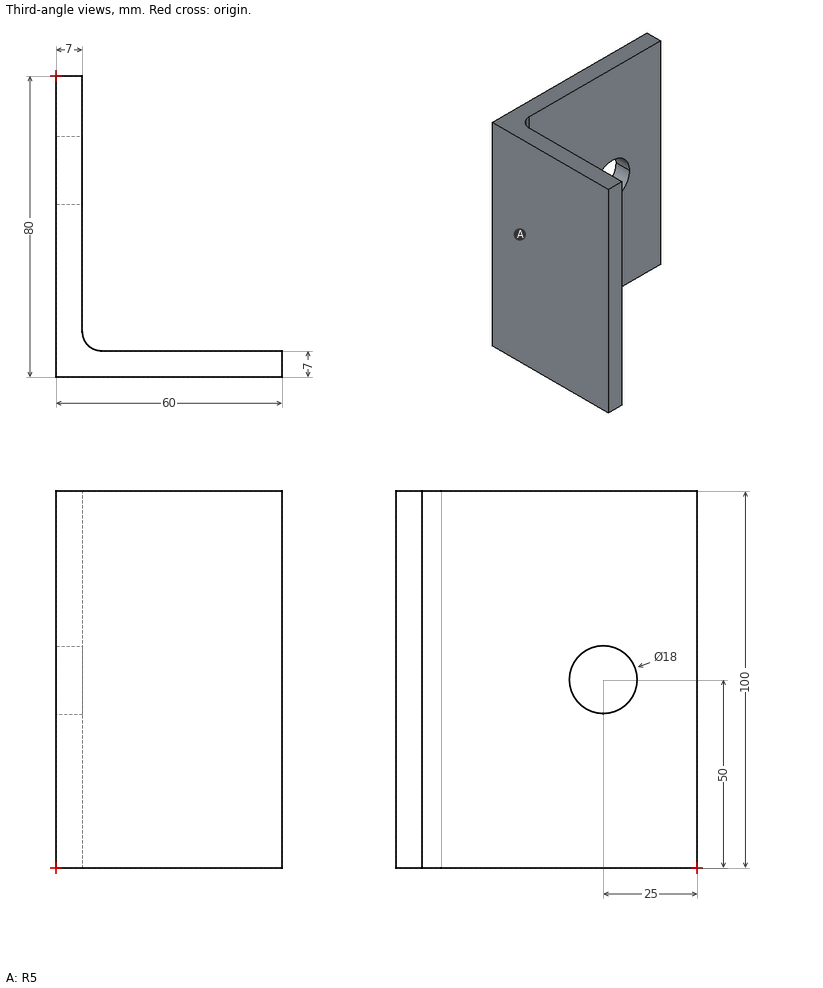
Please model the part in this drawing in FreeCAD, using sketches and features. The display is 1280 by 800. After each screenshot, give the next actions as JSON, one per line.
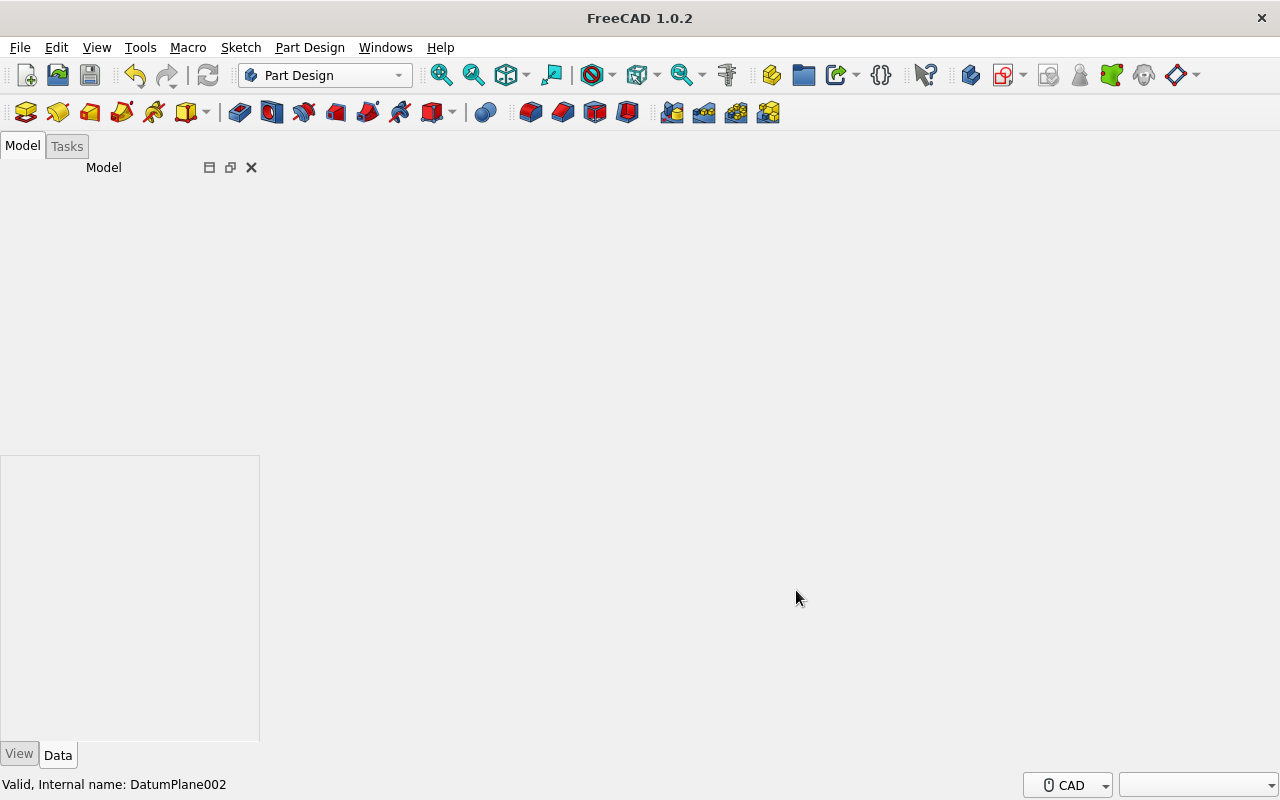
{"action": "key", "text": "ctrl+n"}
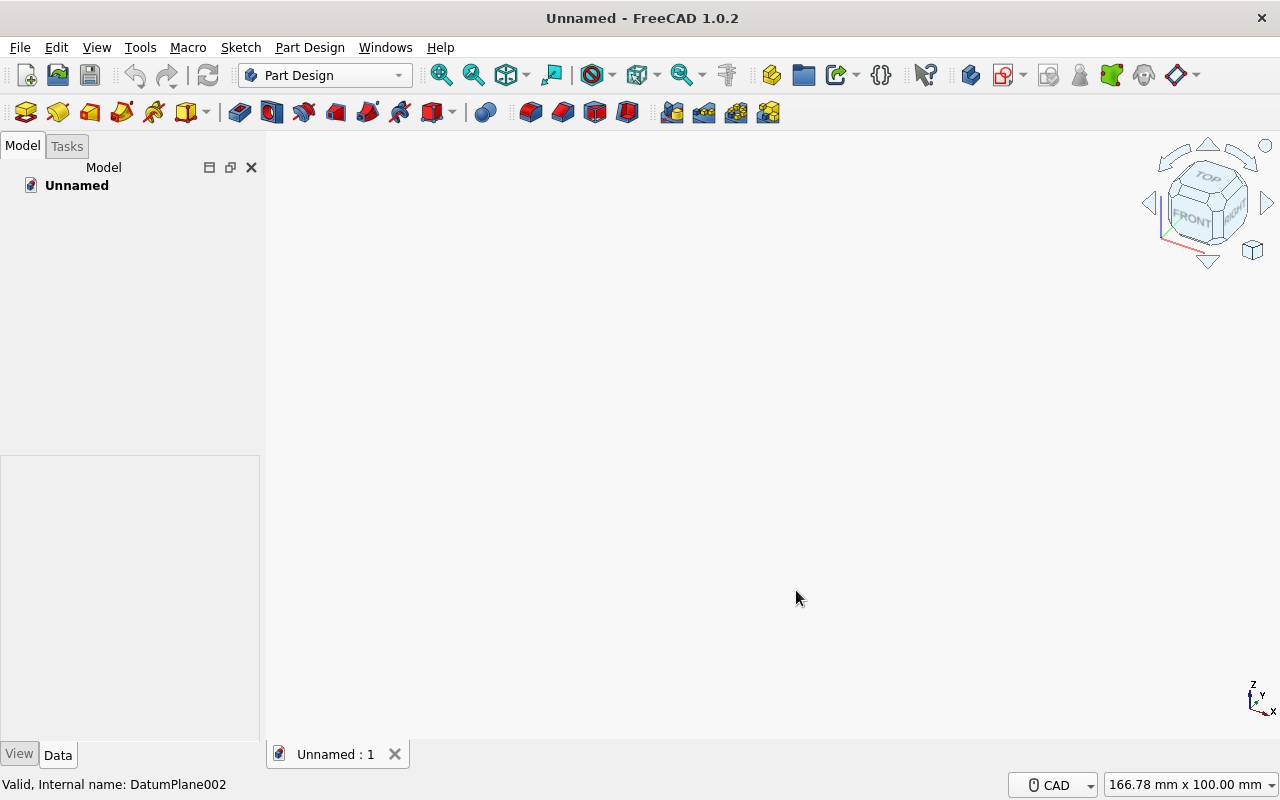
{"action": "left_click", "coordinate": [1004, 76]}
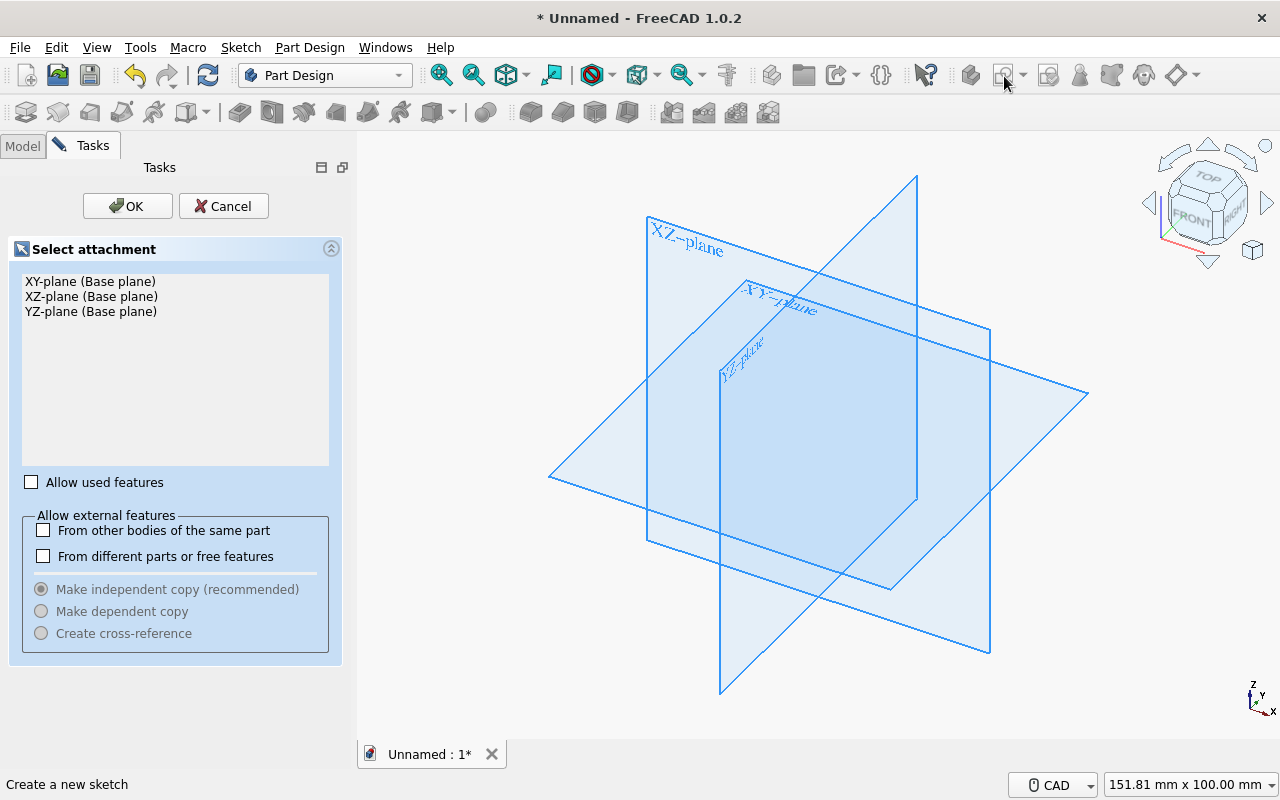
{"action": "left_click", "coordinate": [82, 282]}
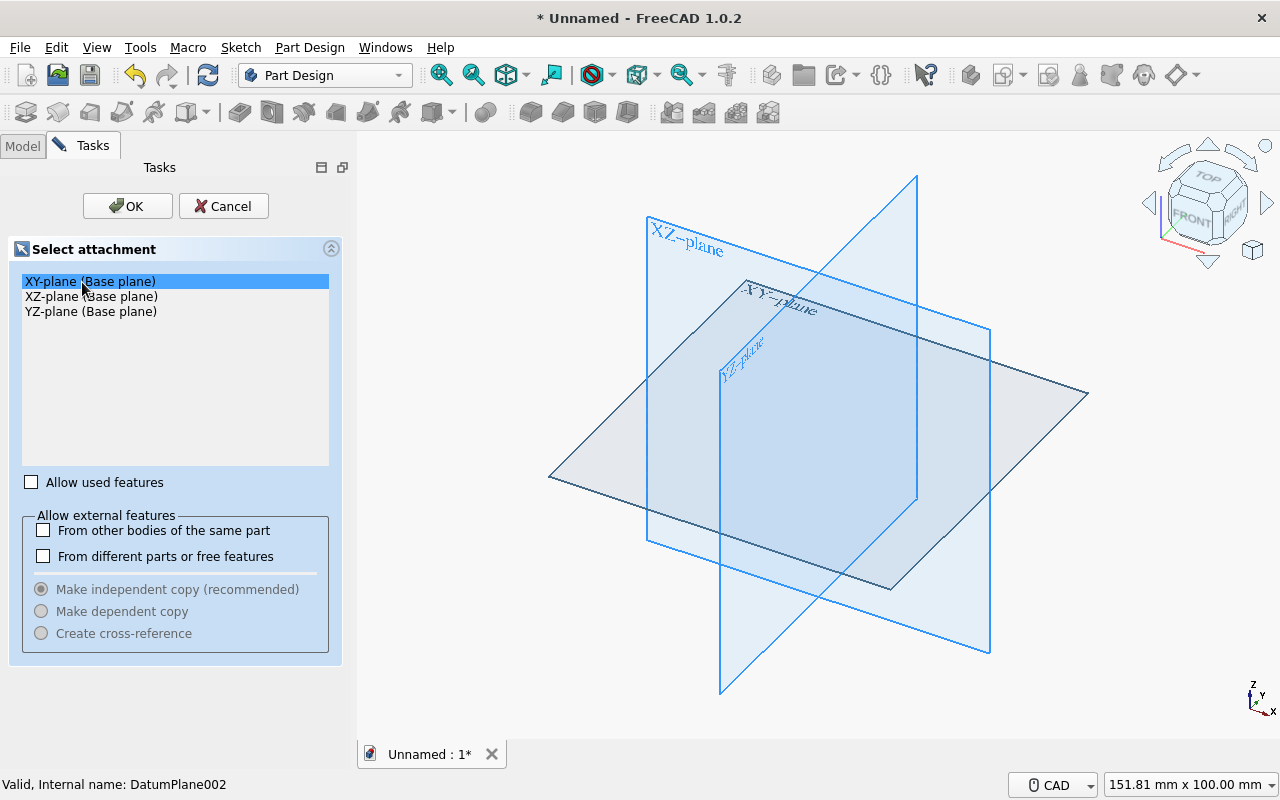
{"action": "left_click", "coordinate": [128, 206]}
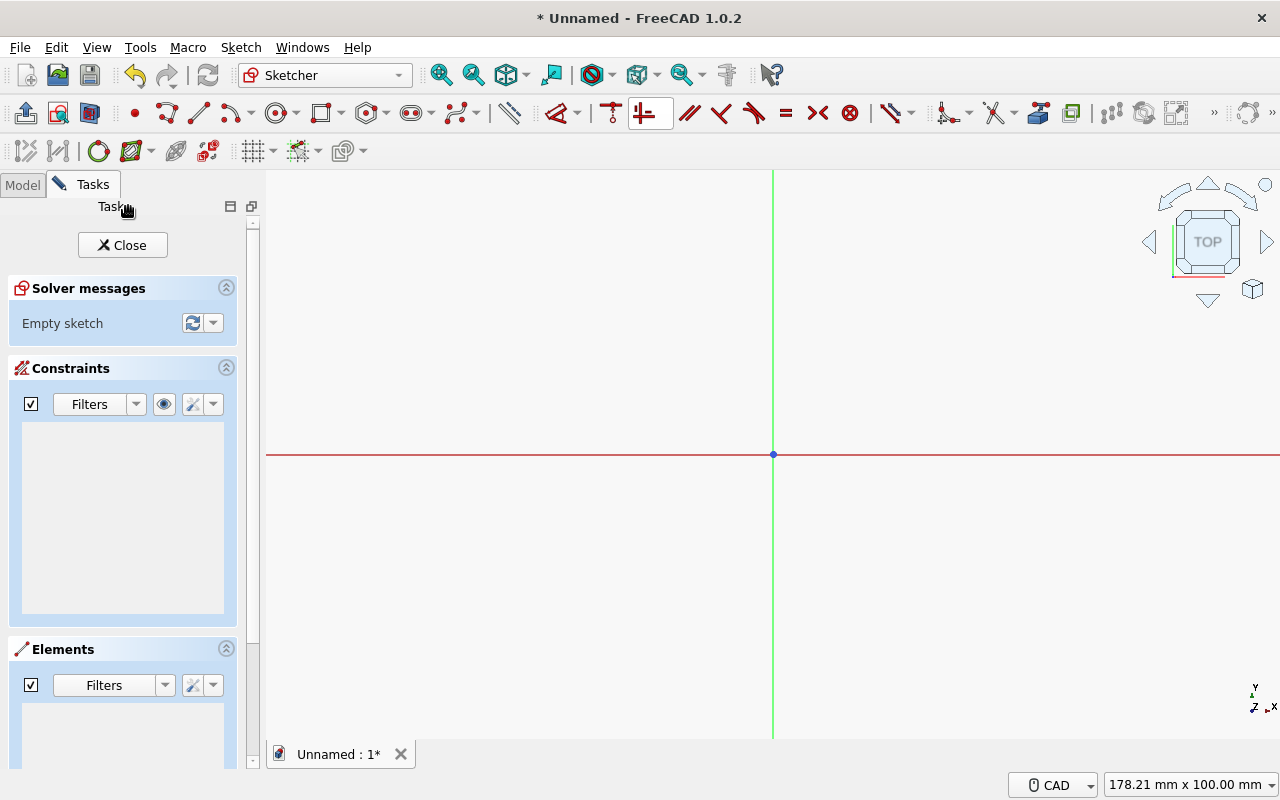
{"action": "scroll", "coordinate": [294, 198], "scroll_direction": "down", "scroll_amount": 2}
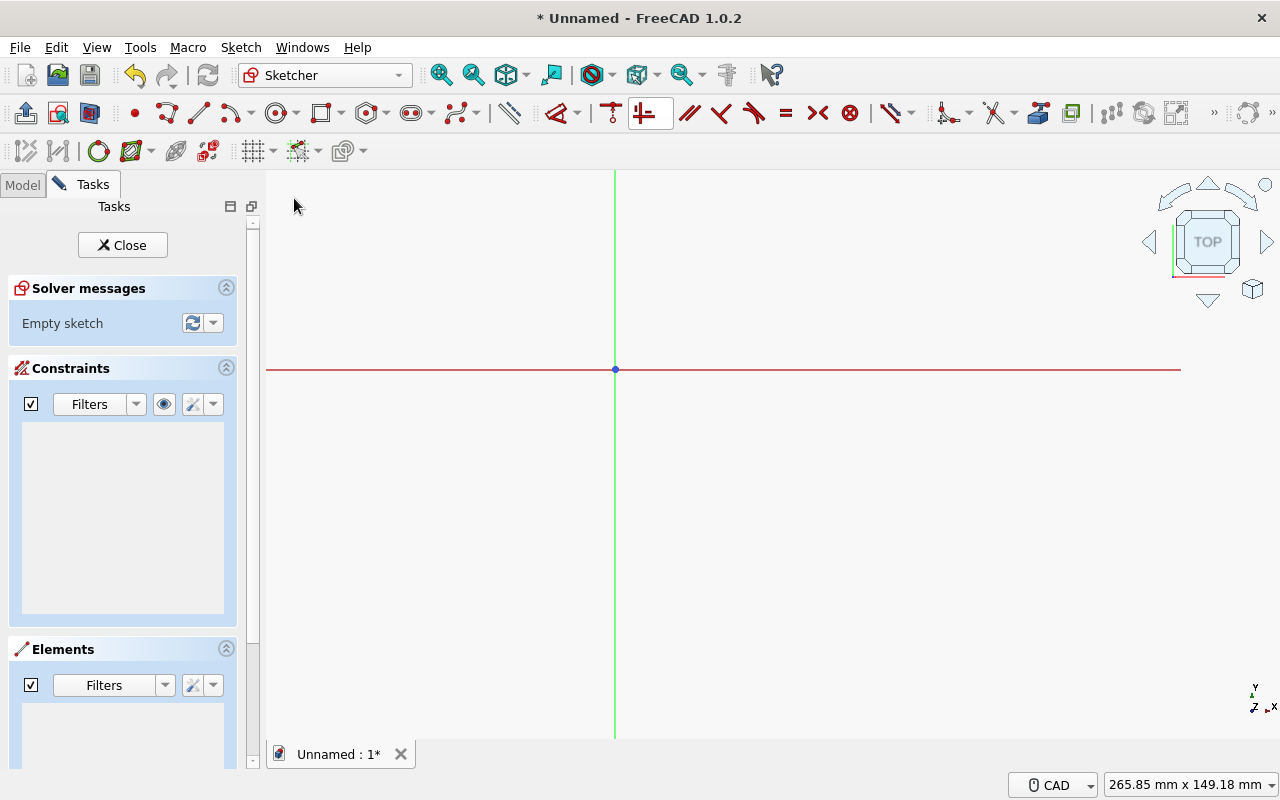
{"action": "key", "text": "g m"}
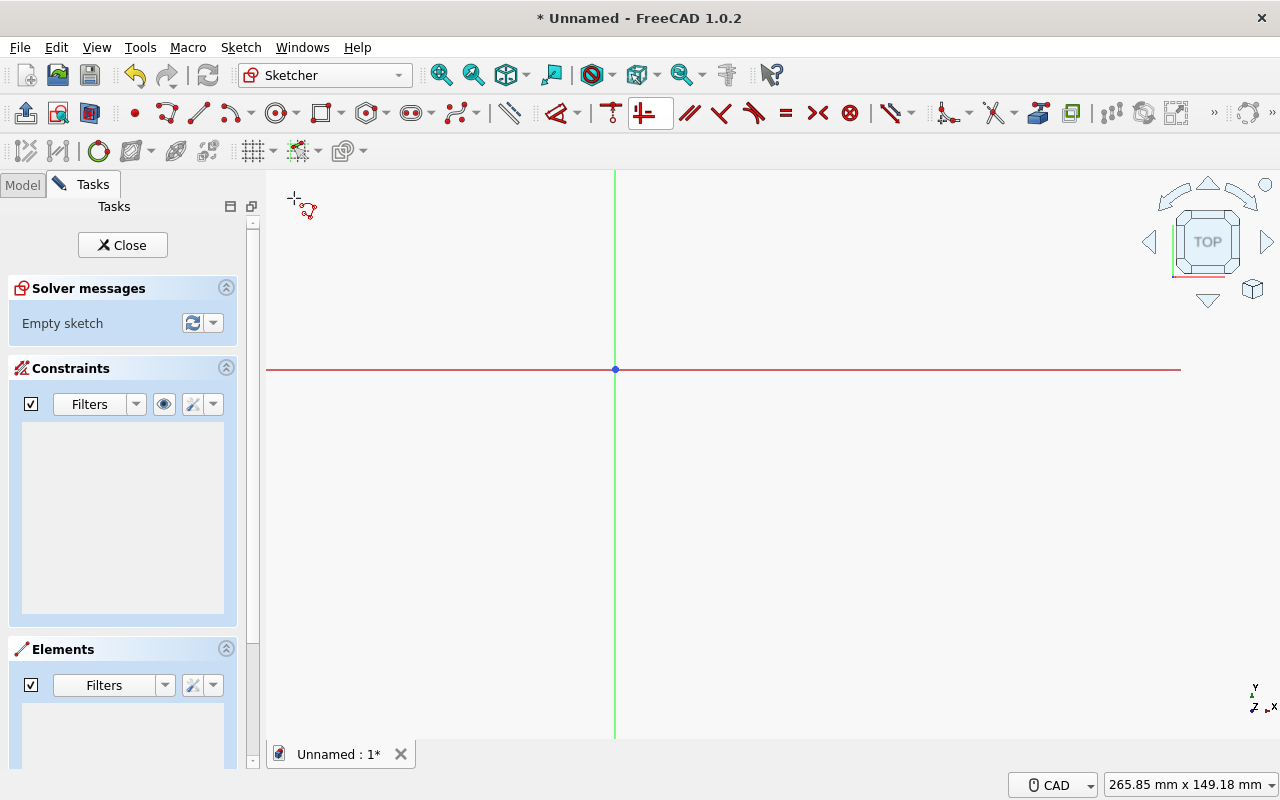
{"action": "left_click", "coordinate": [615, 370]}
{"action": "left_click", "coordinate": [624, 675]}
{"action": "left_click", "coordinate": [844, 675]}
{"action": "left_click", "coordinate": [844, 648]}
{"action": "left_click", "coordinate": [642, 648]}
{"action": "left_click", "coordinate": [642, 379]}
{"action": "left_click", "coordinate": [615, 370]}
{"action": "key", "text": "Escape"}
{"action": "key", "text": "Escape"}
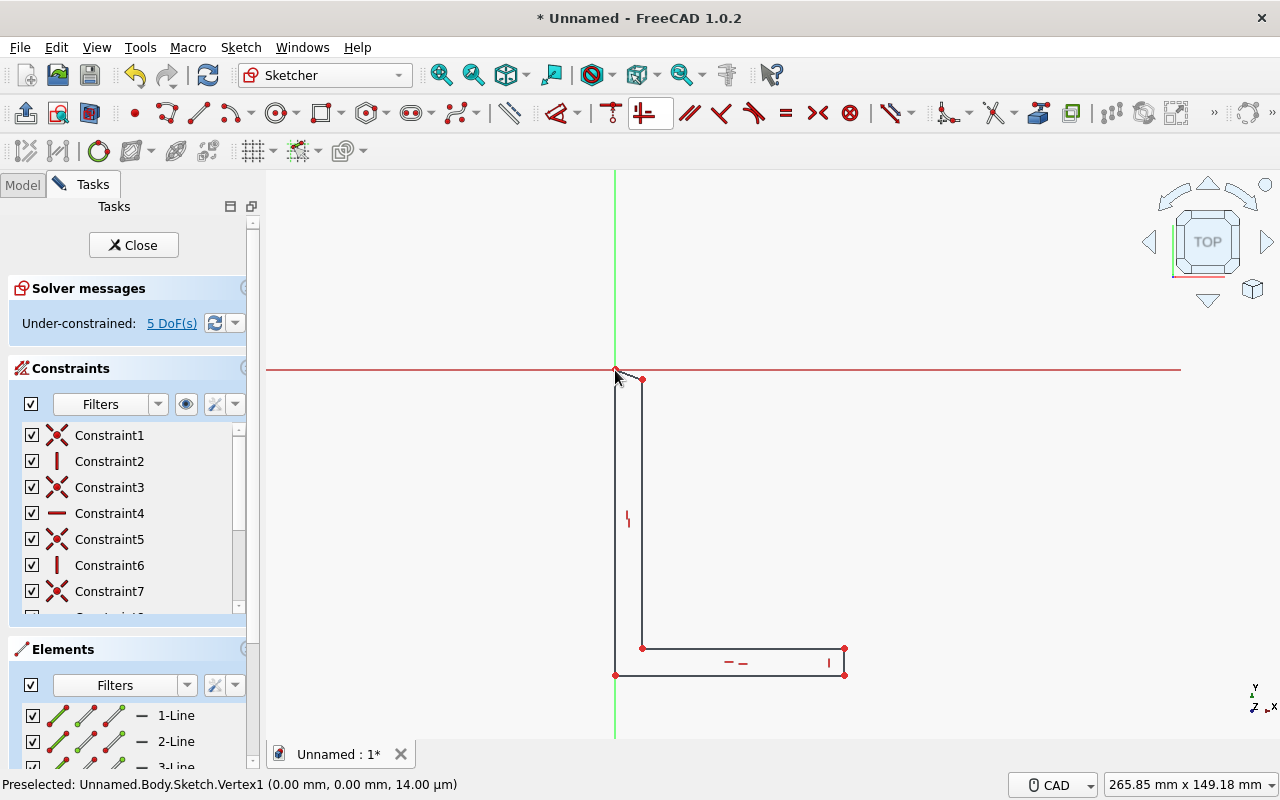
{"action": "scroll", "coordinate": [623, 373], "scroll_direction": "up", "scroll_amount": 3}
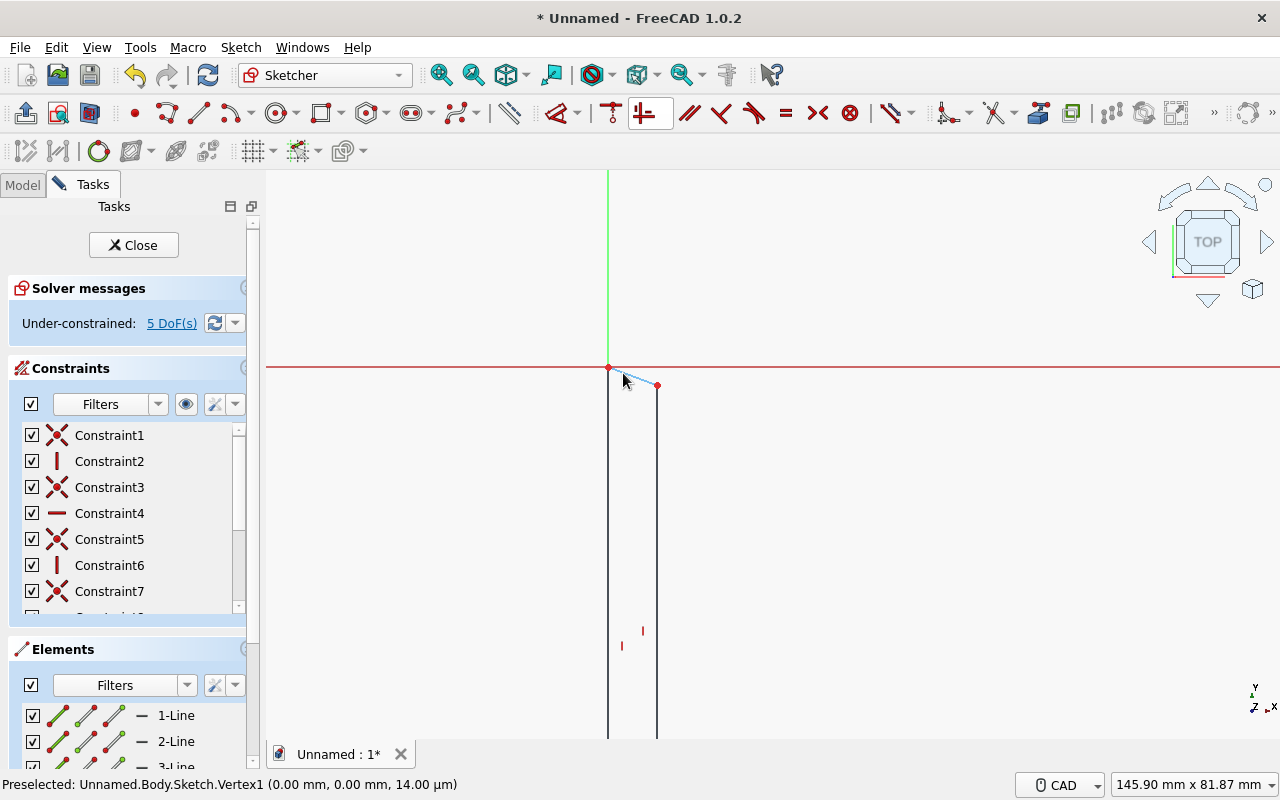
{"action": "left_click", "coordinate": [623, 373]}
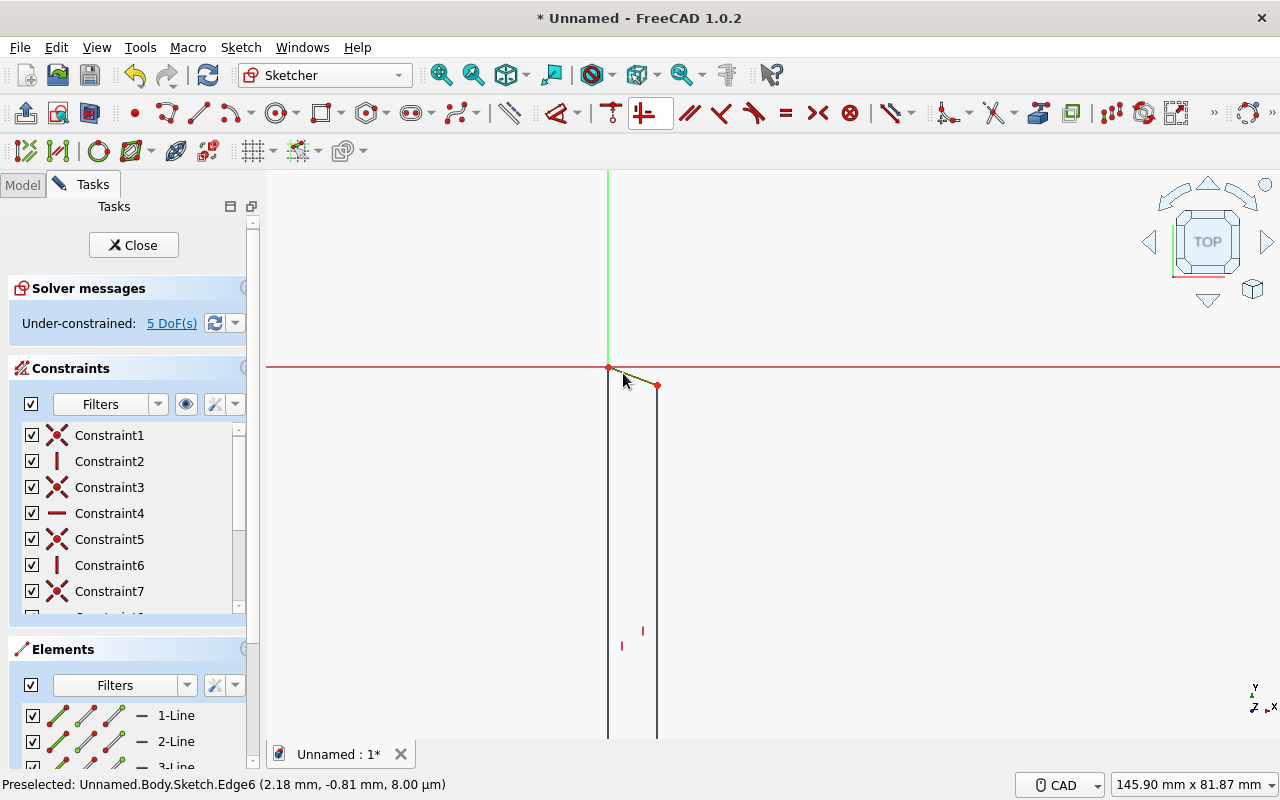
{"action": "key", "text": "h"}